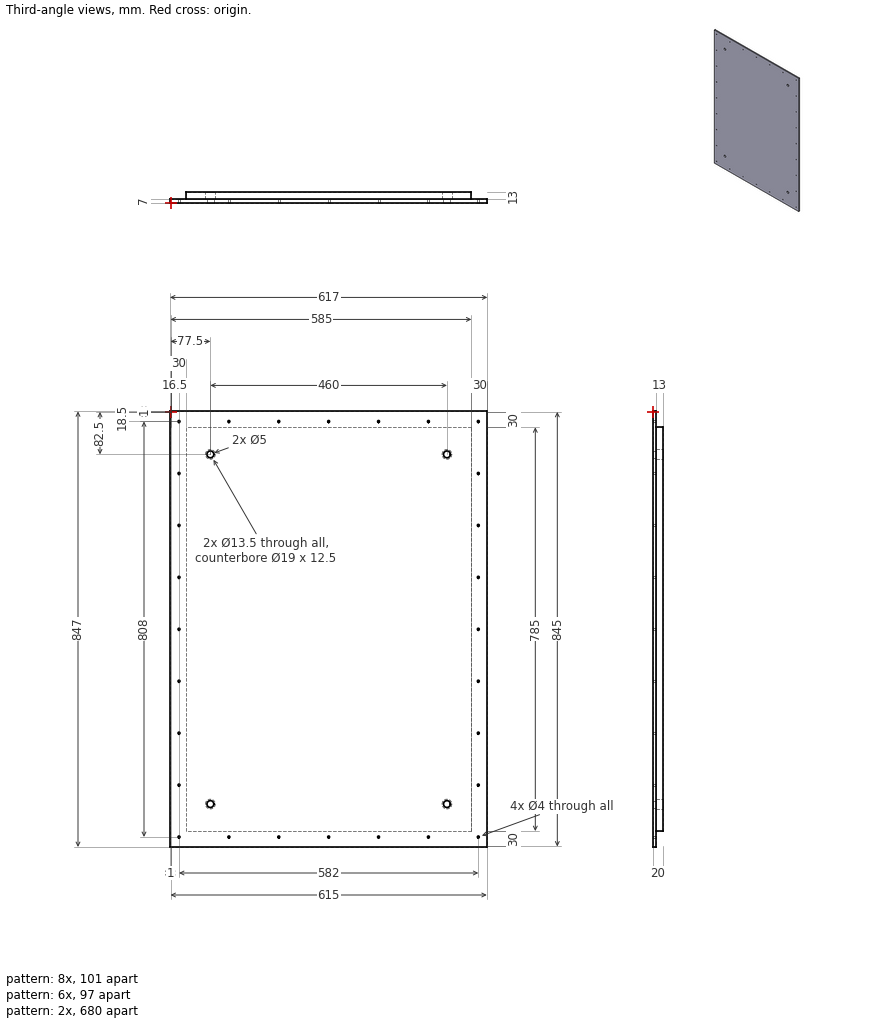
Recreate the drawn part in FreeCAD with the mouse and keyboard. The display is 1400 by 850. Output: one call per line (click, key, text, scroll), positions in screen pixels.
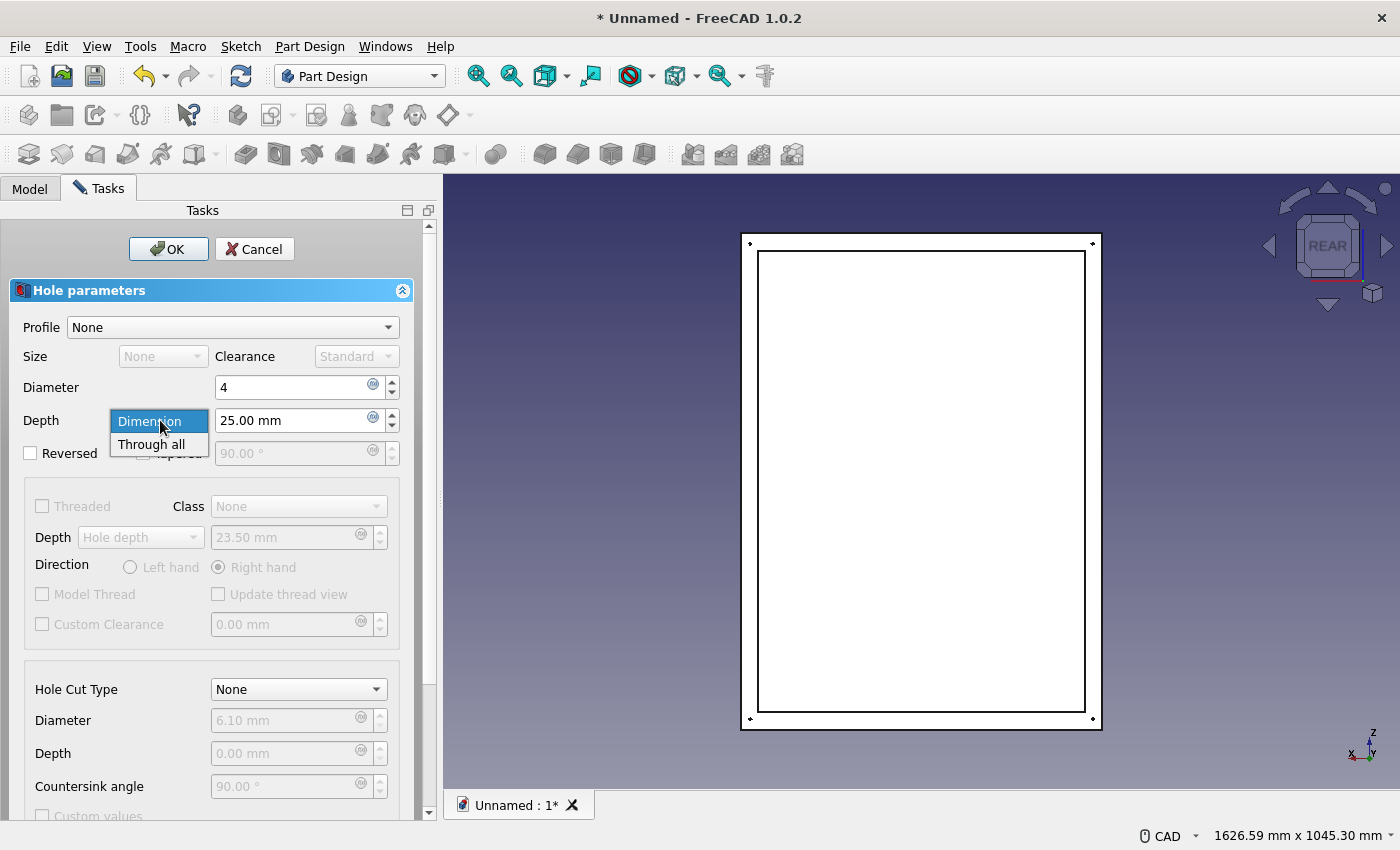
click(158, 444)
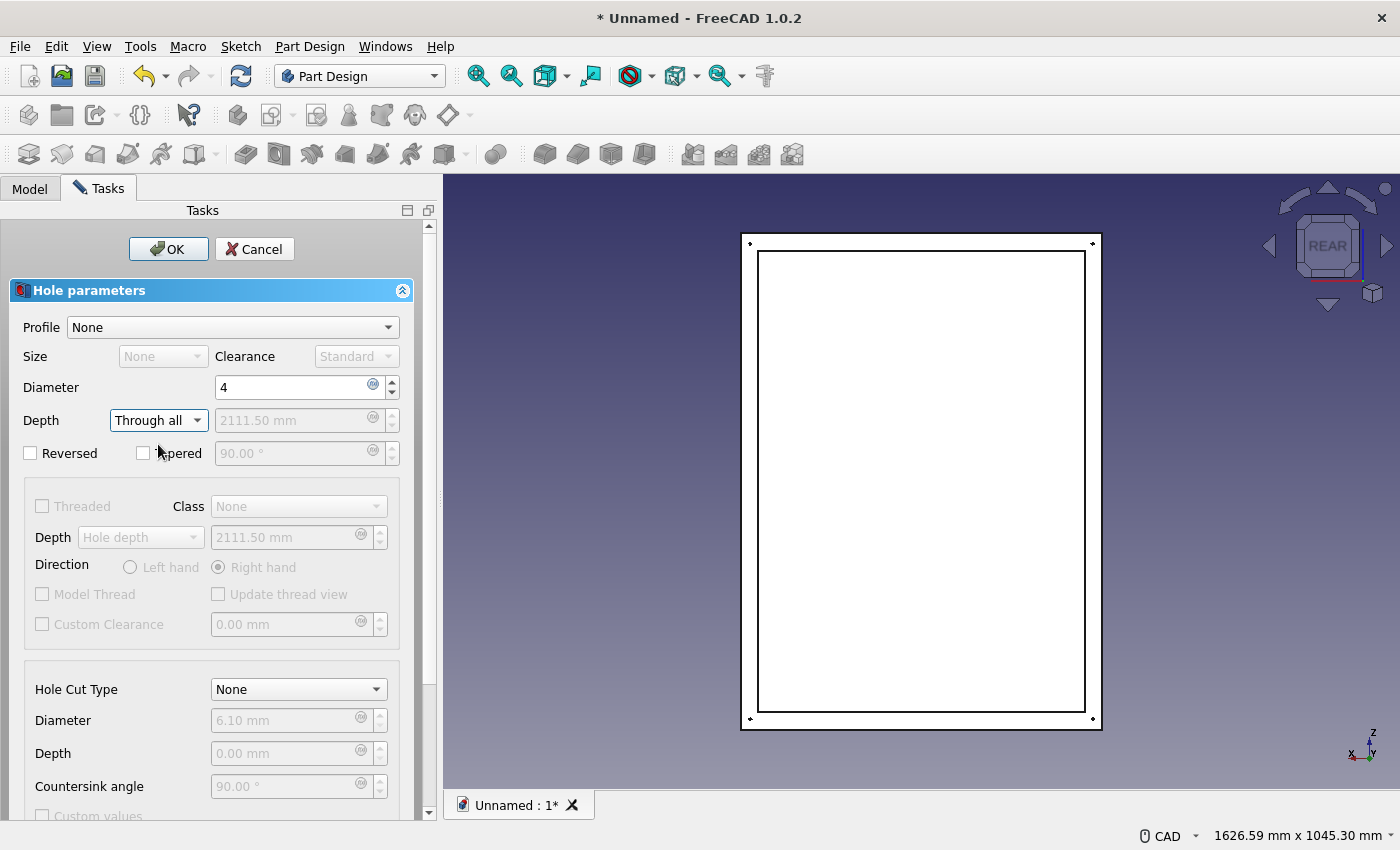
click(169, 249)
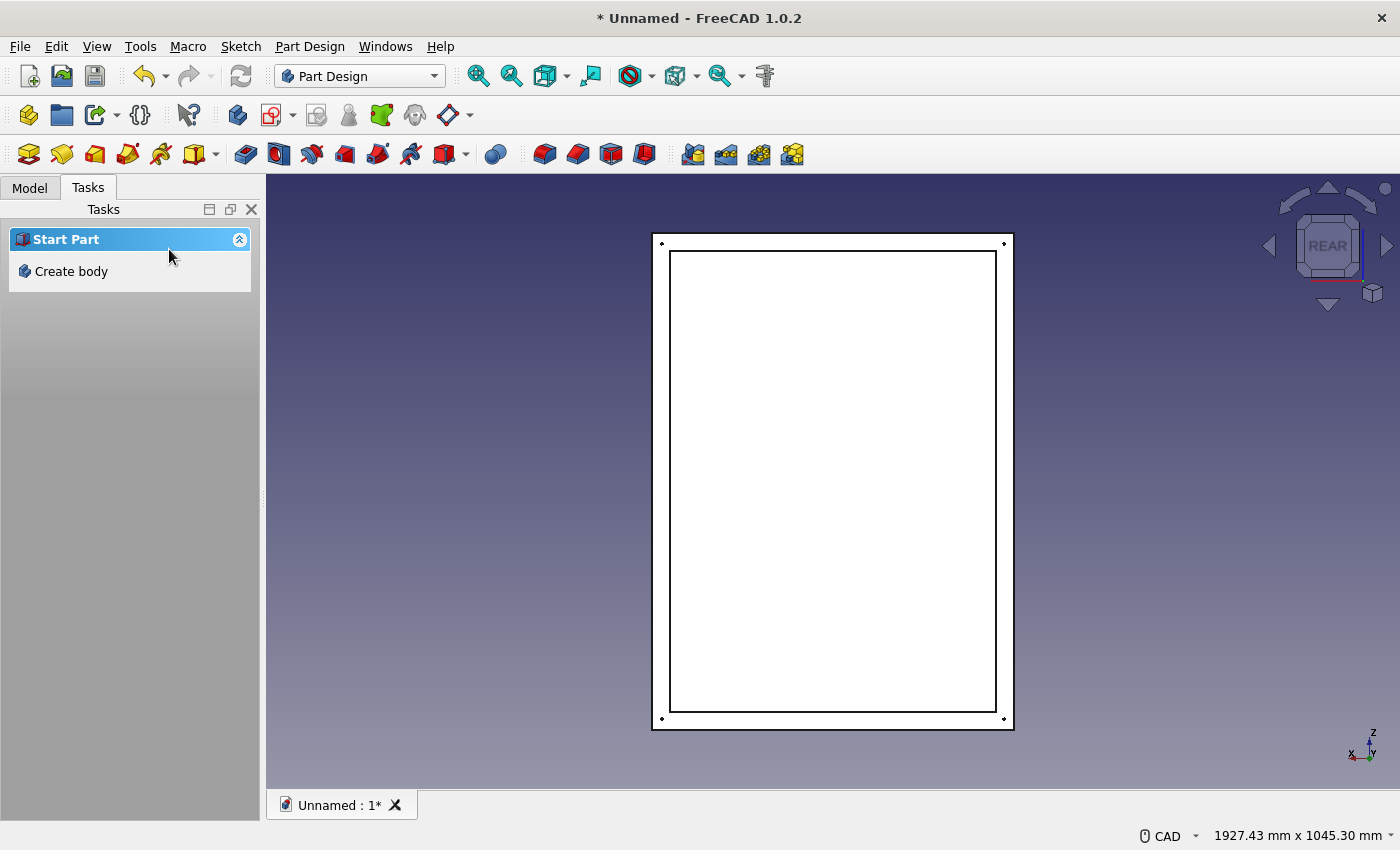
click(30, 188)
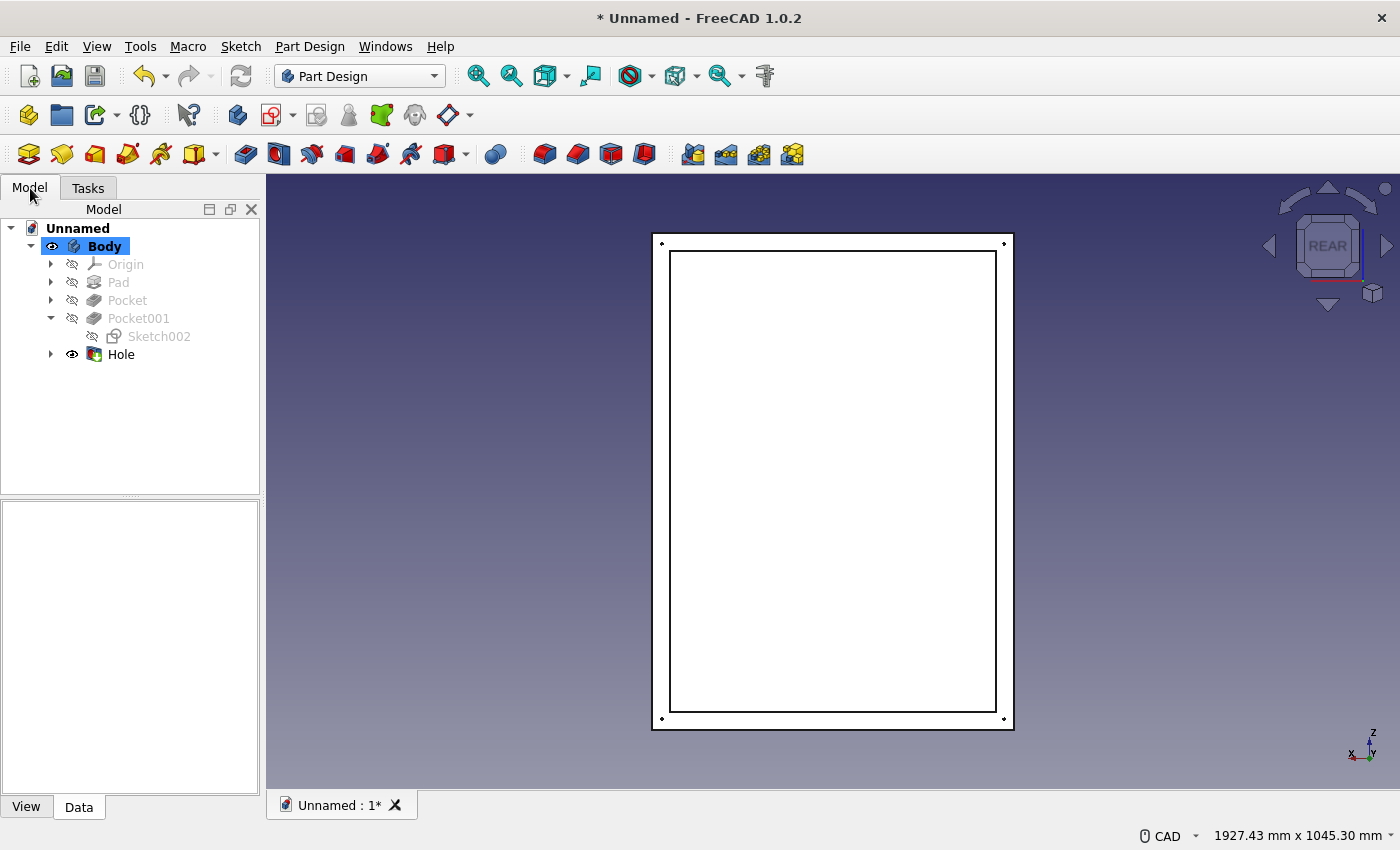
click(117, 354)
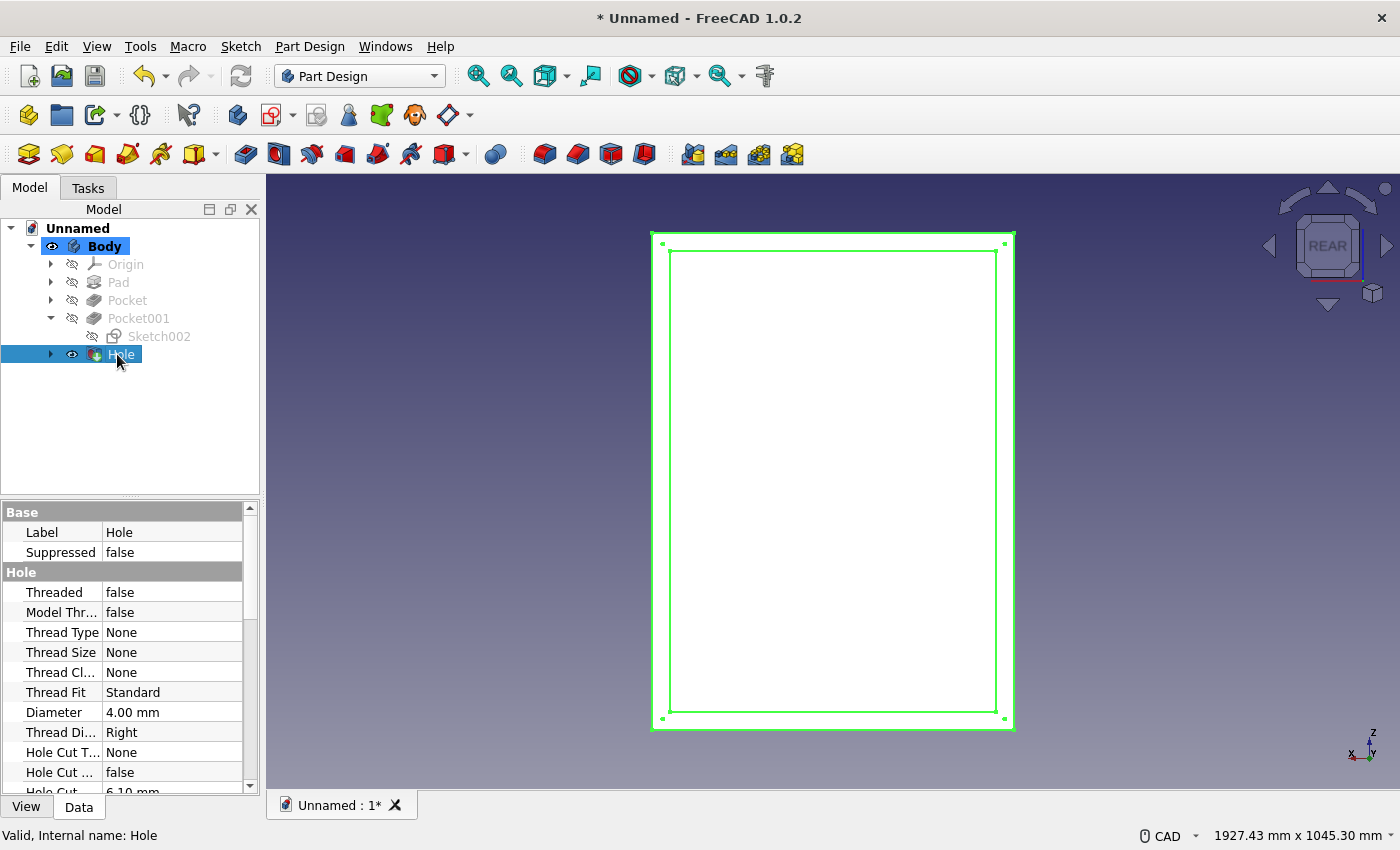
click(726, 154)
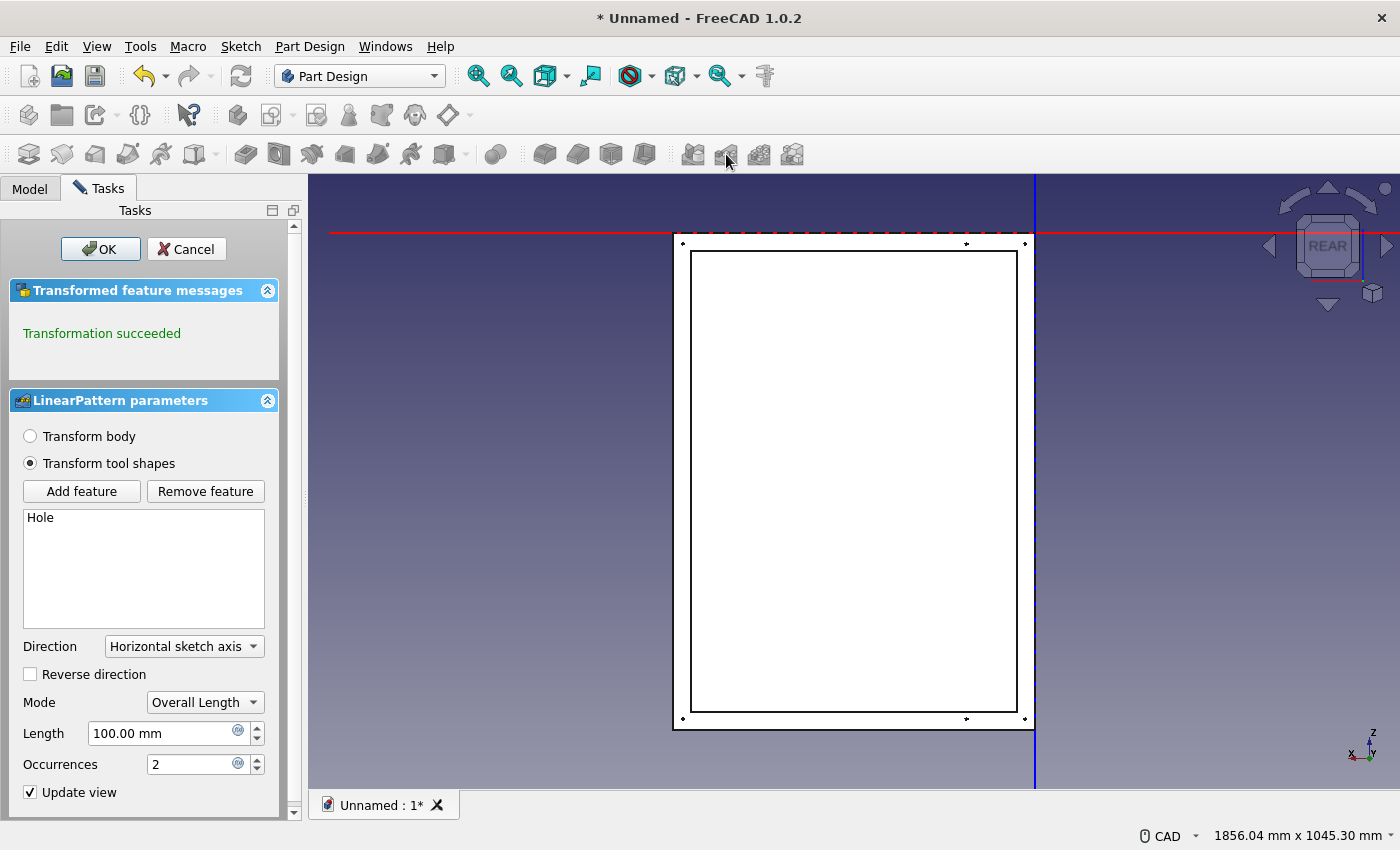
click(185, 646)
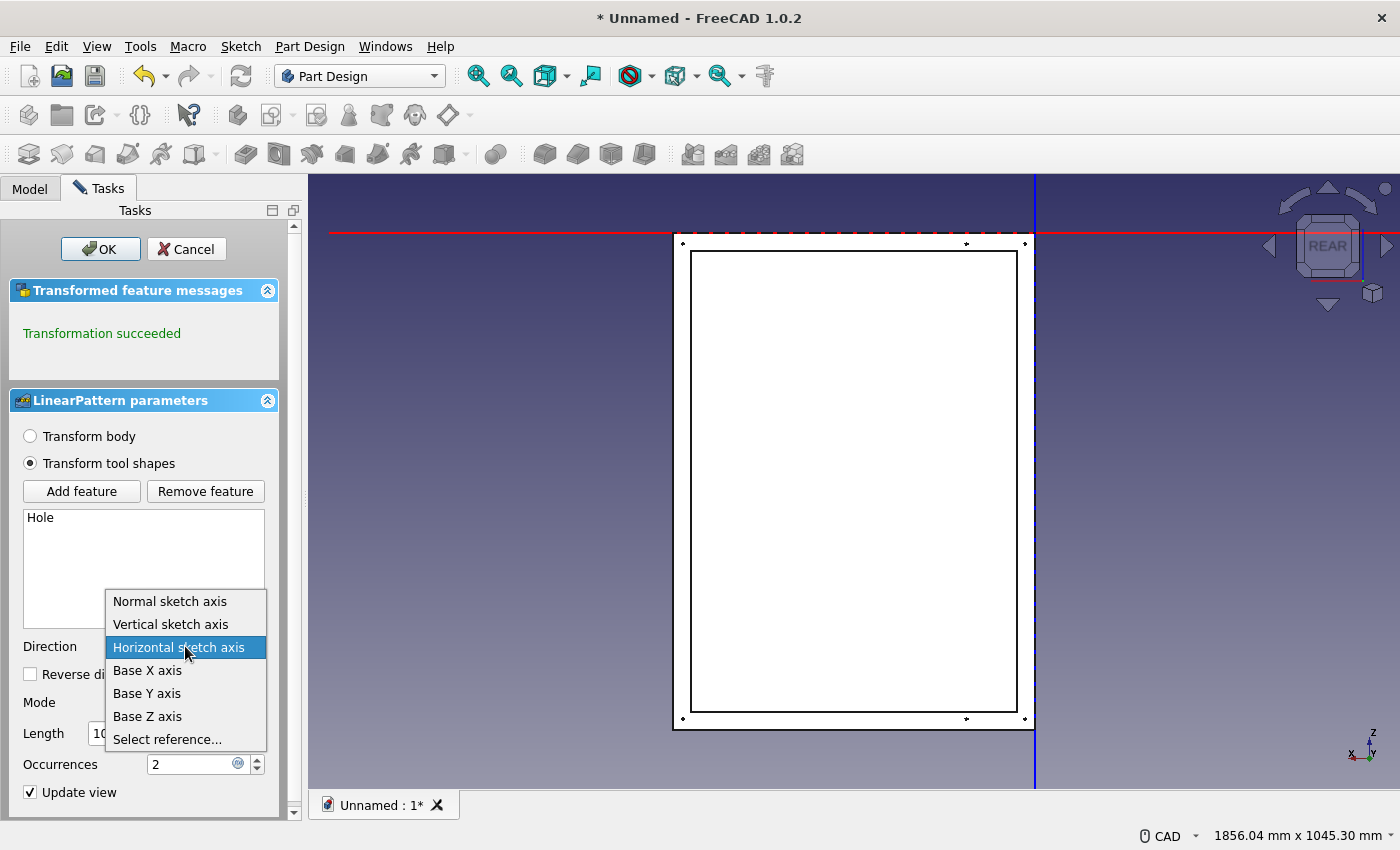
click(184, 716)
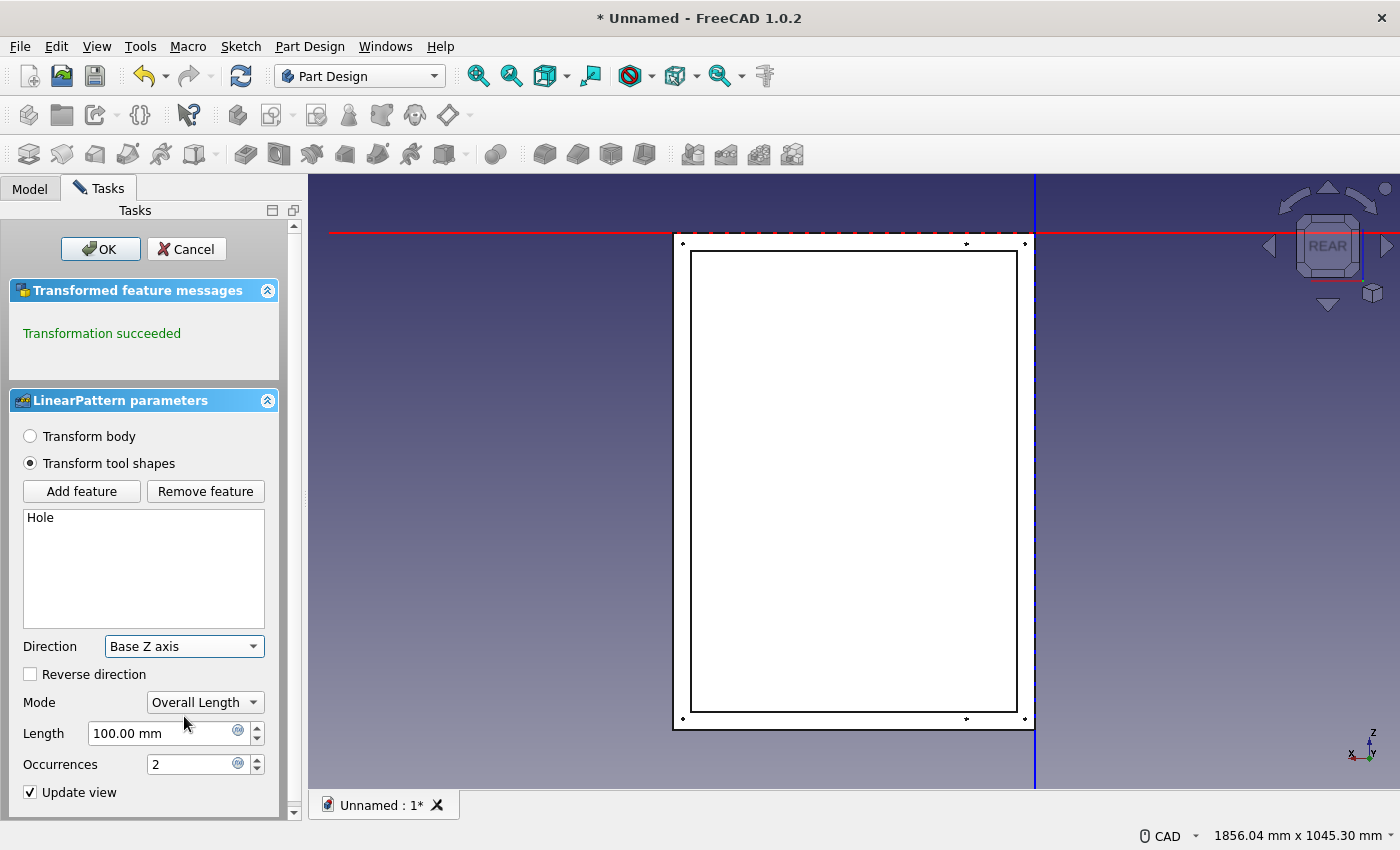
click(206, 702)